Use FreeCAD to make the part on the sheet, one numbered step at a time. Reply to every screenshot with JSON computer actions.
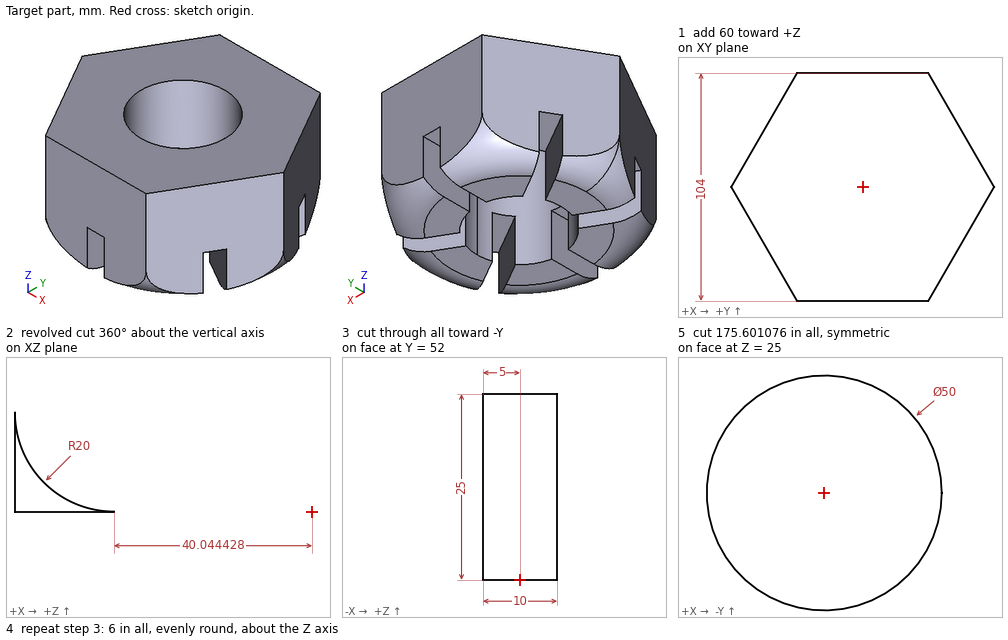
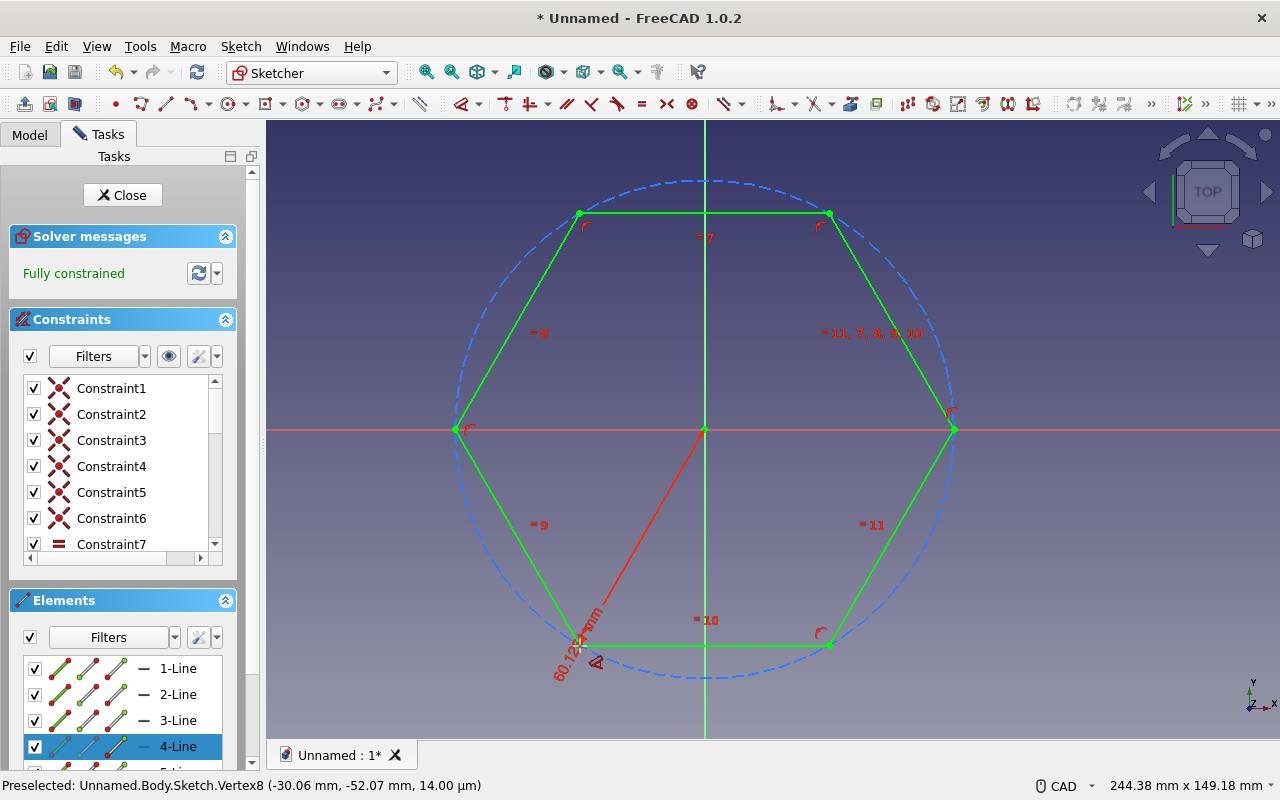
{"action": "left_click", "coordinate": [829, 213]}
{"action": "left_click", "coordinate": [546, 330]}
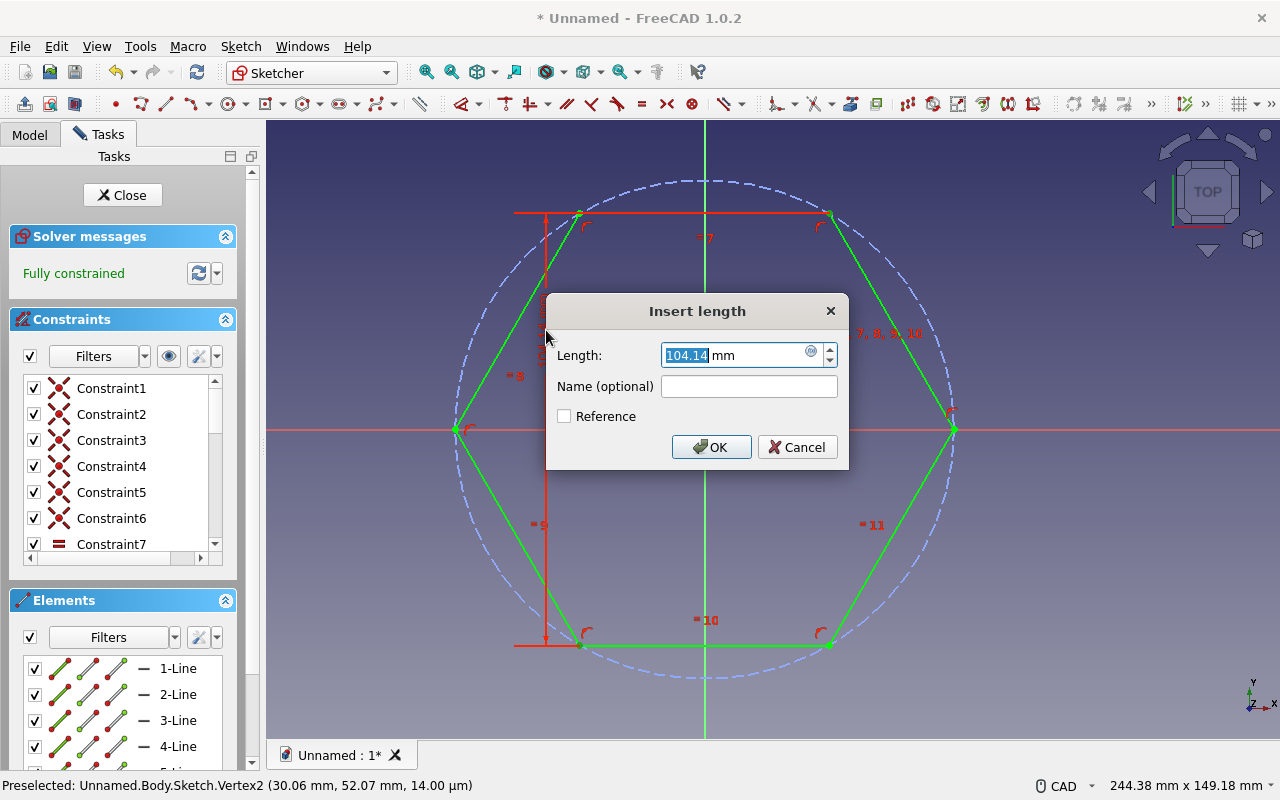
{"action": "type", "text": "104"}
{"action": "key", "text": "Return"}
{"action": "key", "text": "Escape"}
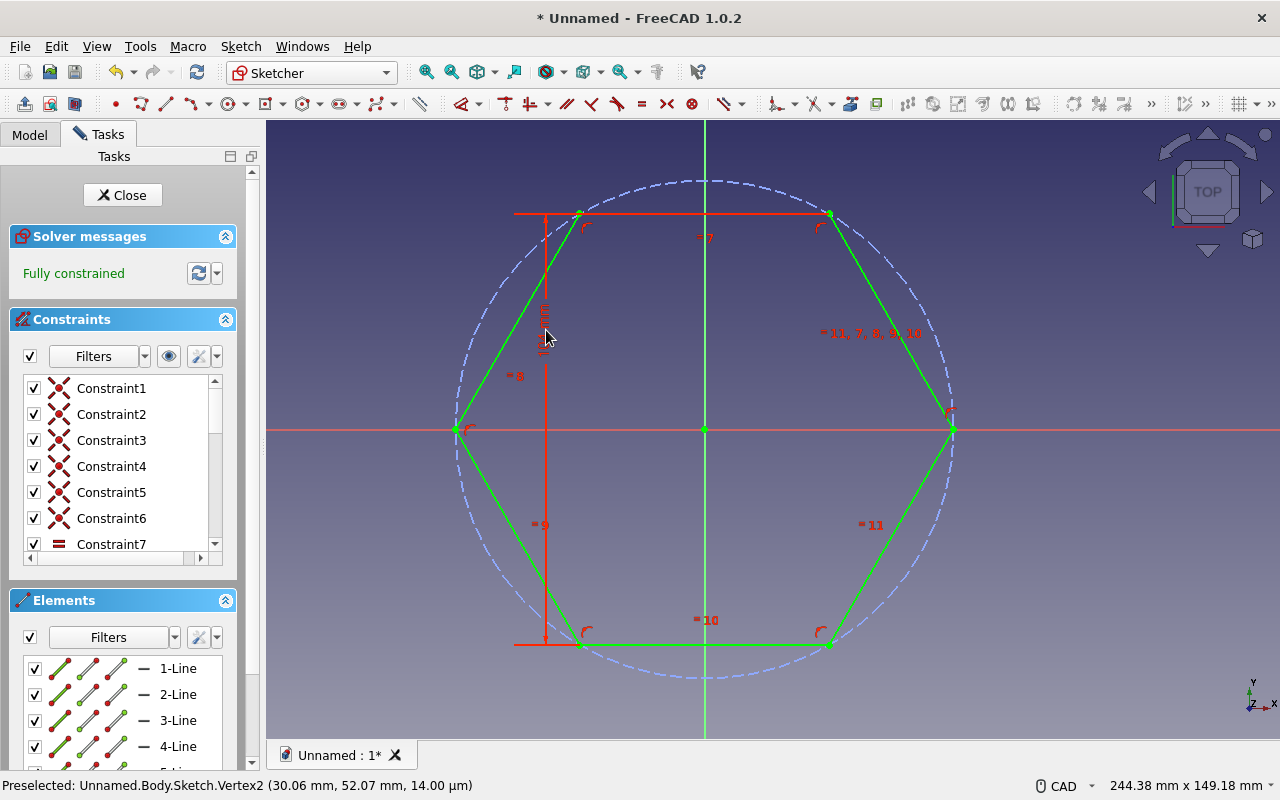
{"action": "left_click", "coordinate": [123, 195]}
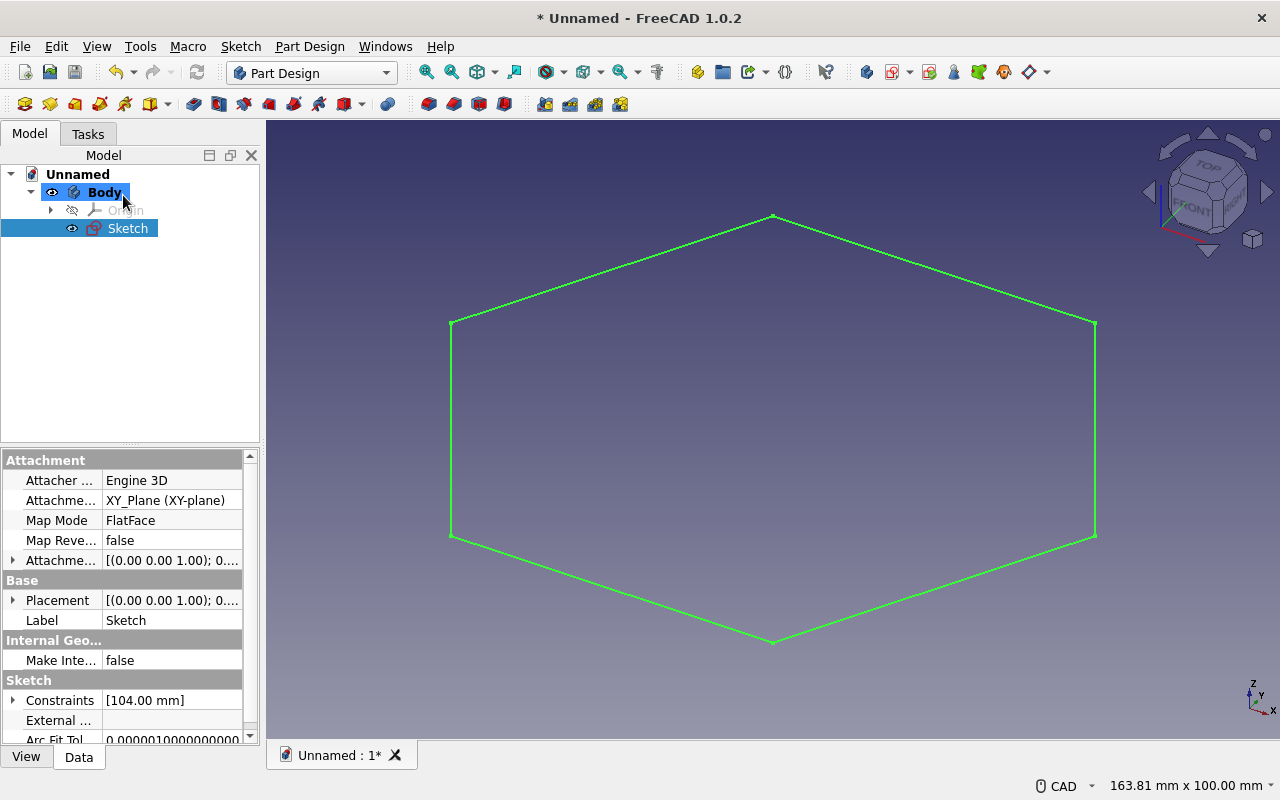
{"action": "left_click", "coordinate": [25, 104]}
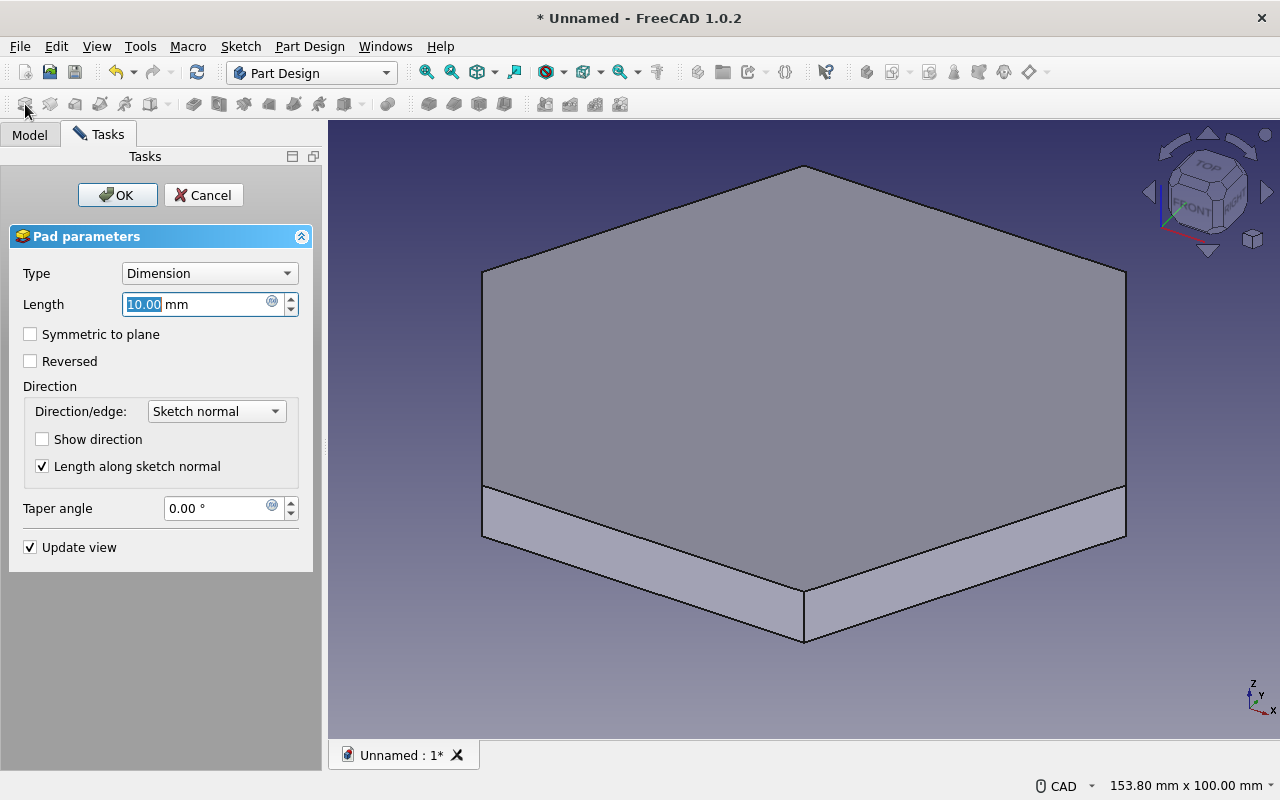
{"action": "type", "text": "60"}
{"action": "key", "text": "Tab"}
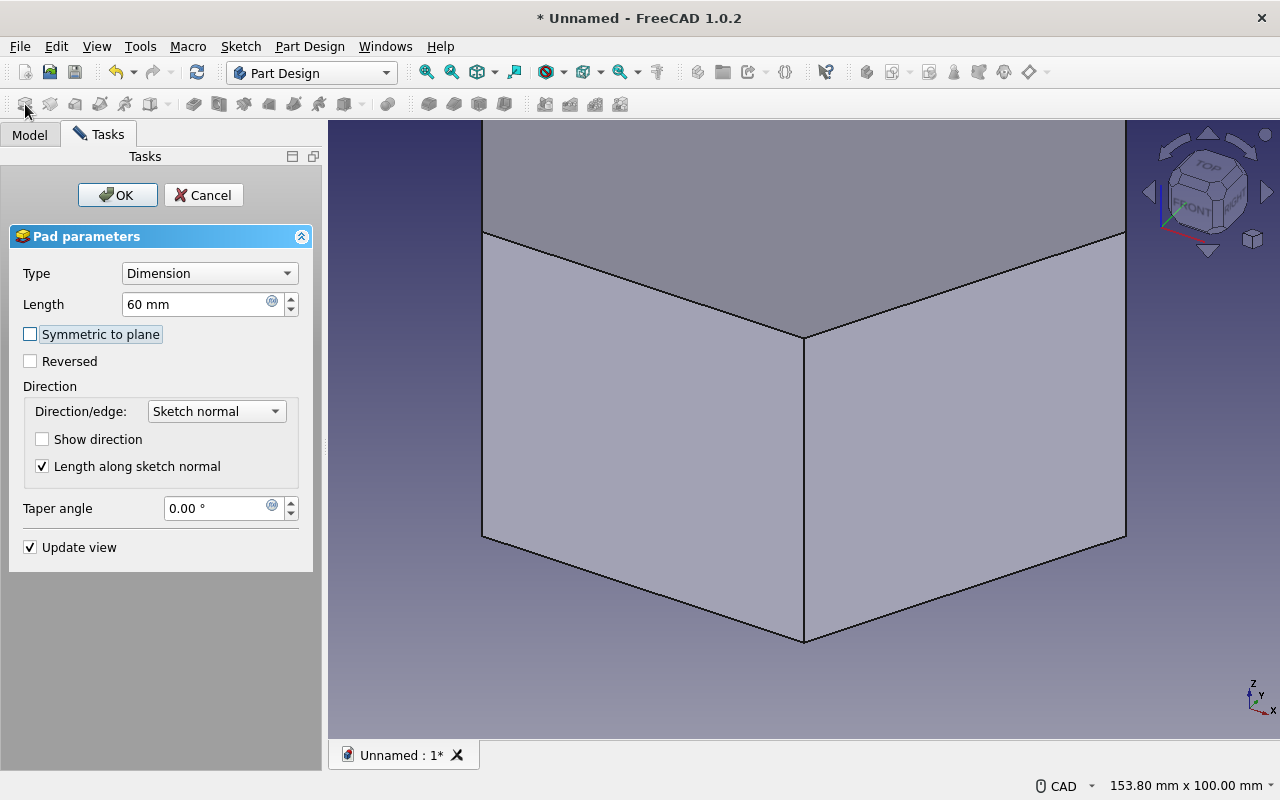
{"action": "left_click", "coordinate": [118, 195]}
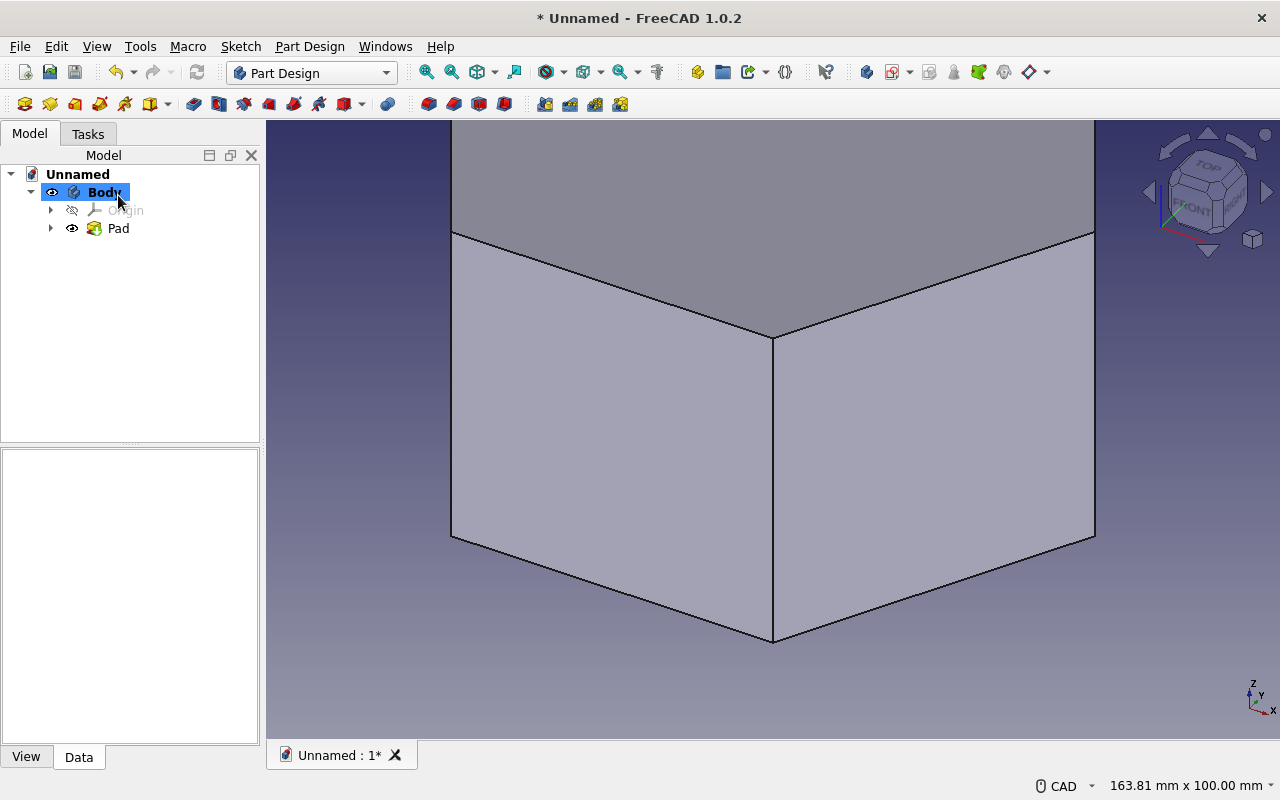
{"action": "left_click", "coordinate": [427, 72]}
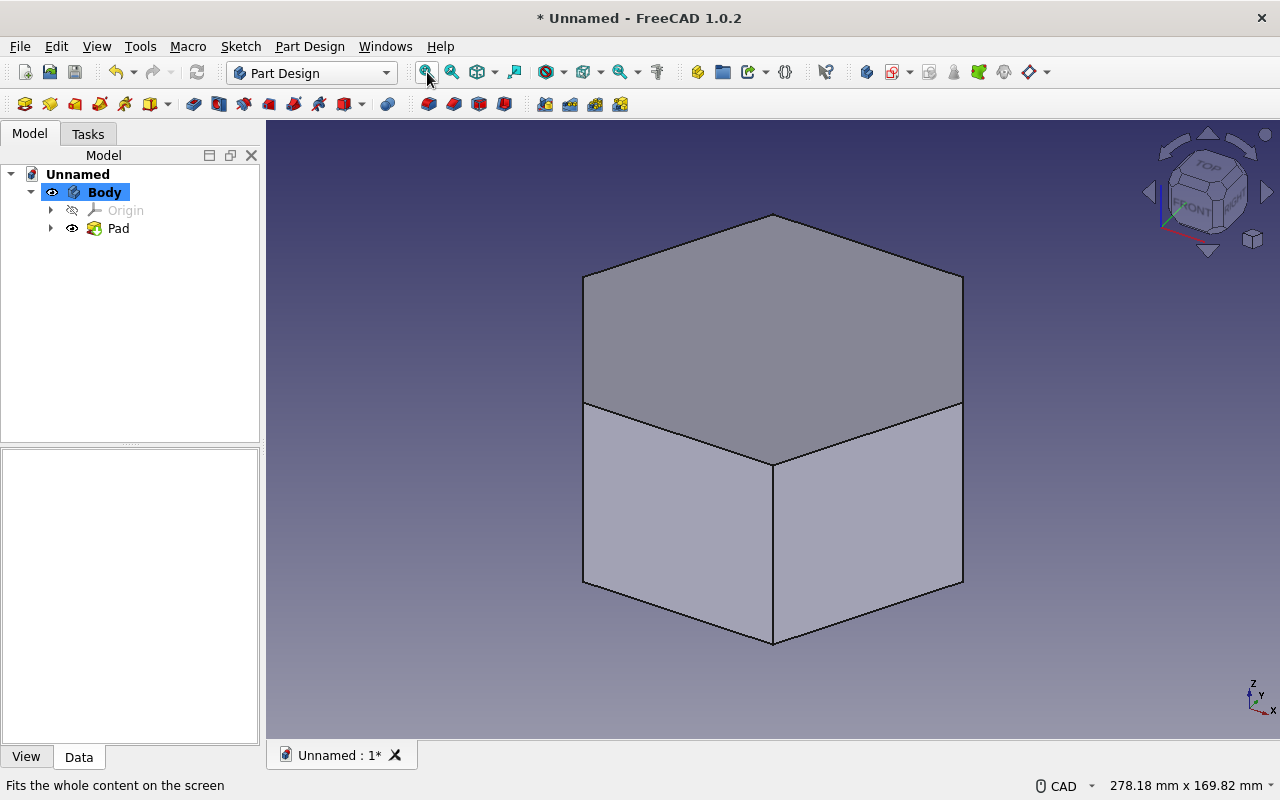
{"action": "left_click", "coordinate": [892, 72]}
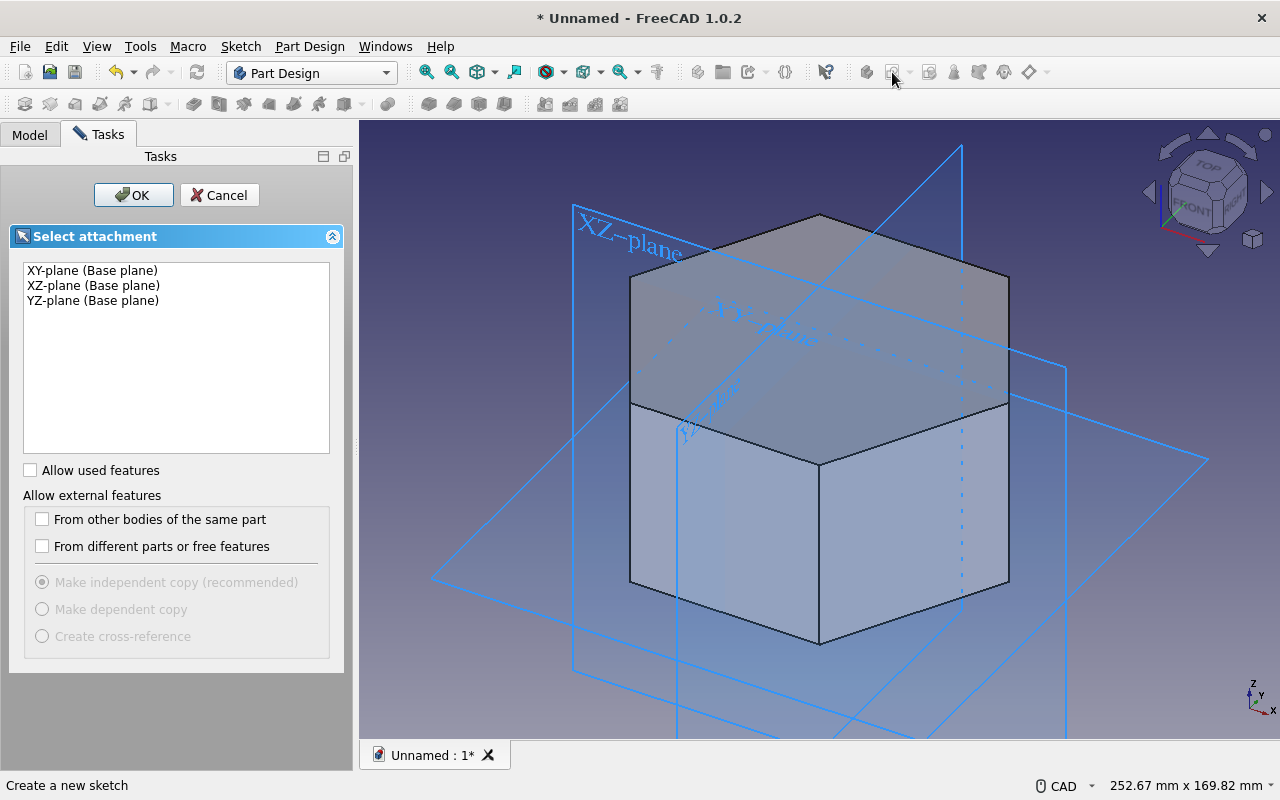
{"action": "left_click", "coordinate": [84, 286]}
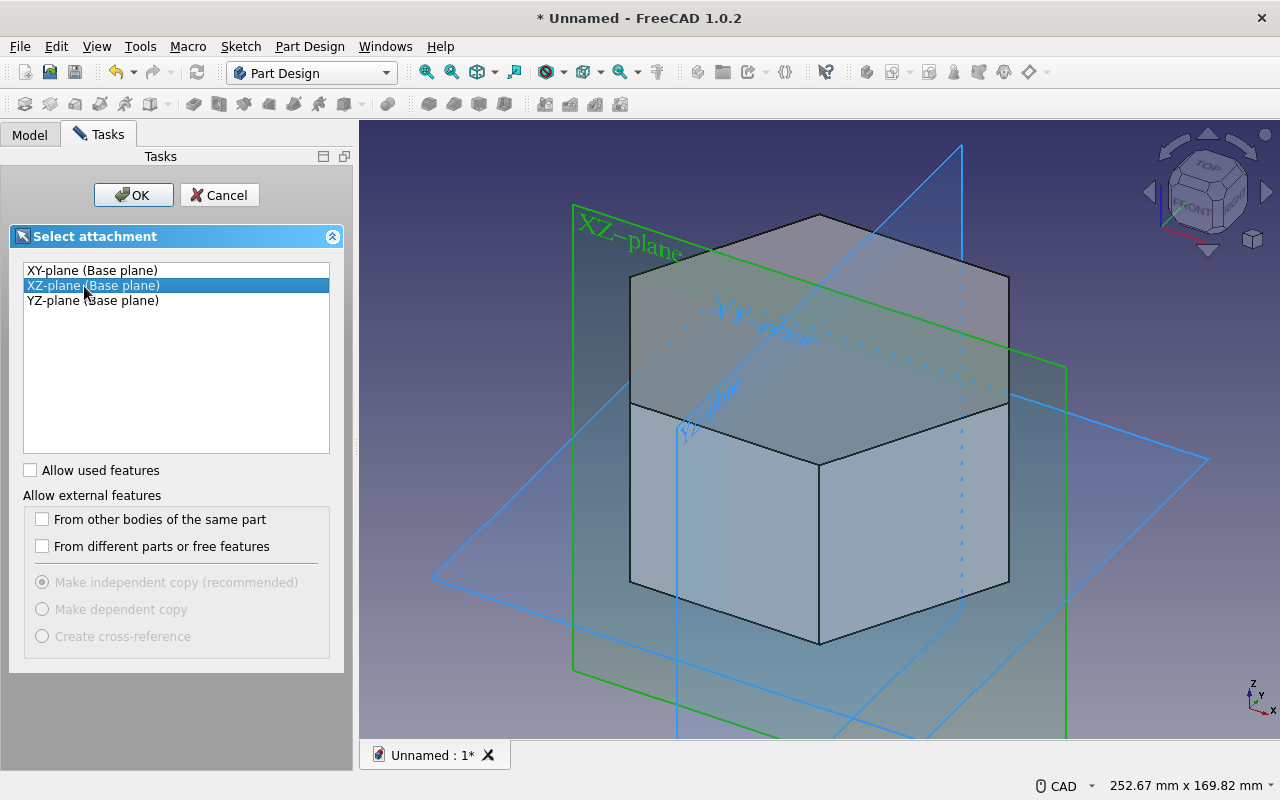
{"action": "left_click", "coordinate": [134, 195]}